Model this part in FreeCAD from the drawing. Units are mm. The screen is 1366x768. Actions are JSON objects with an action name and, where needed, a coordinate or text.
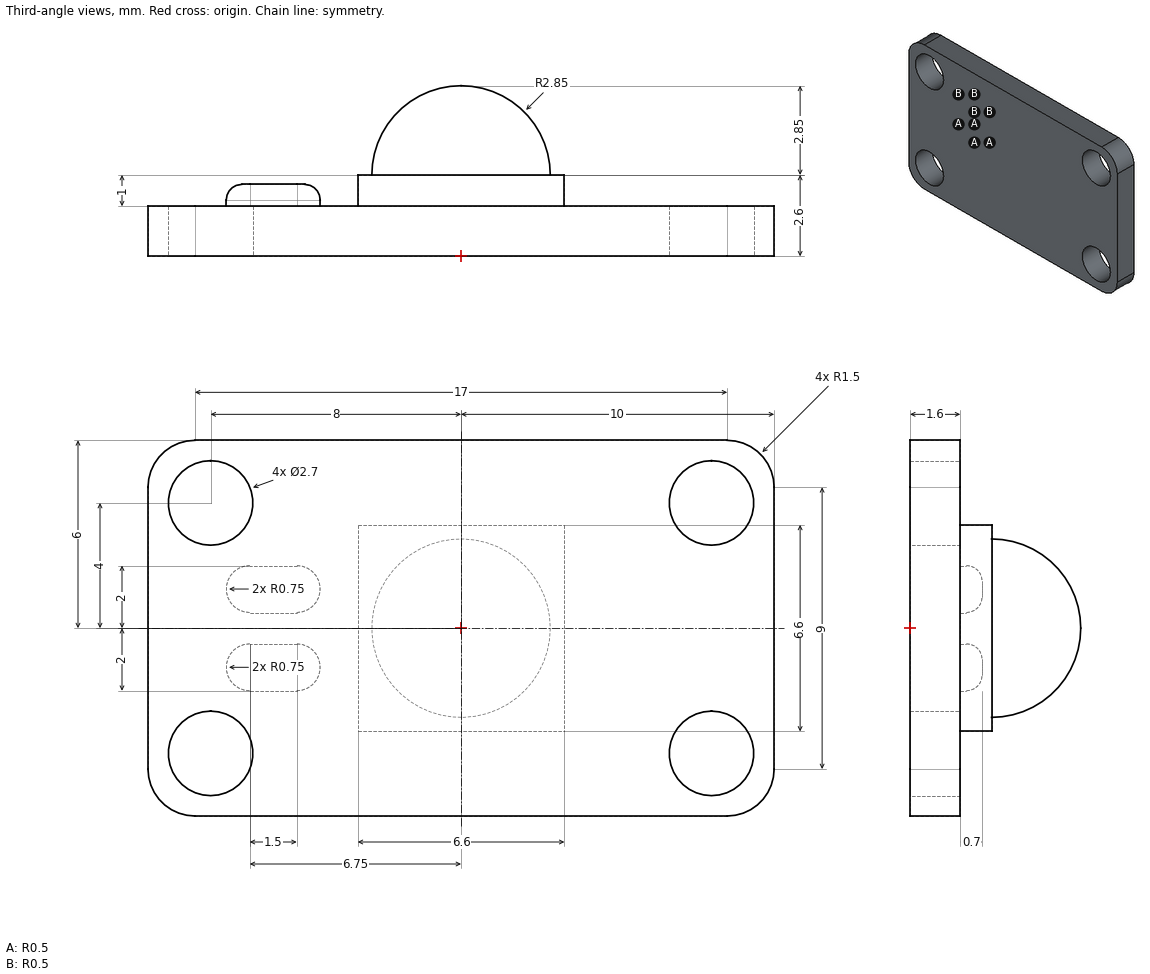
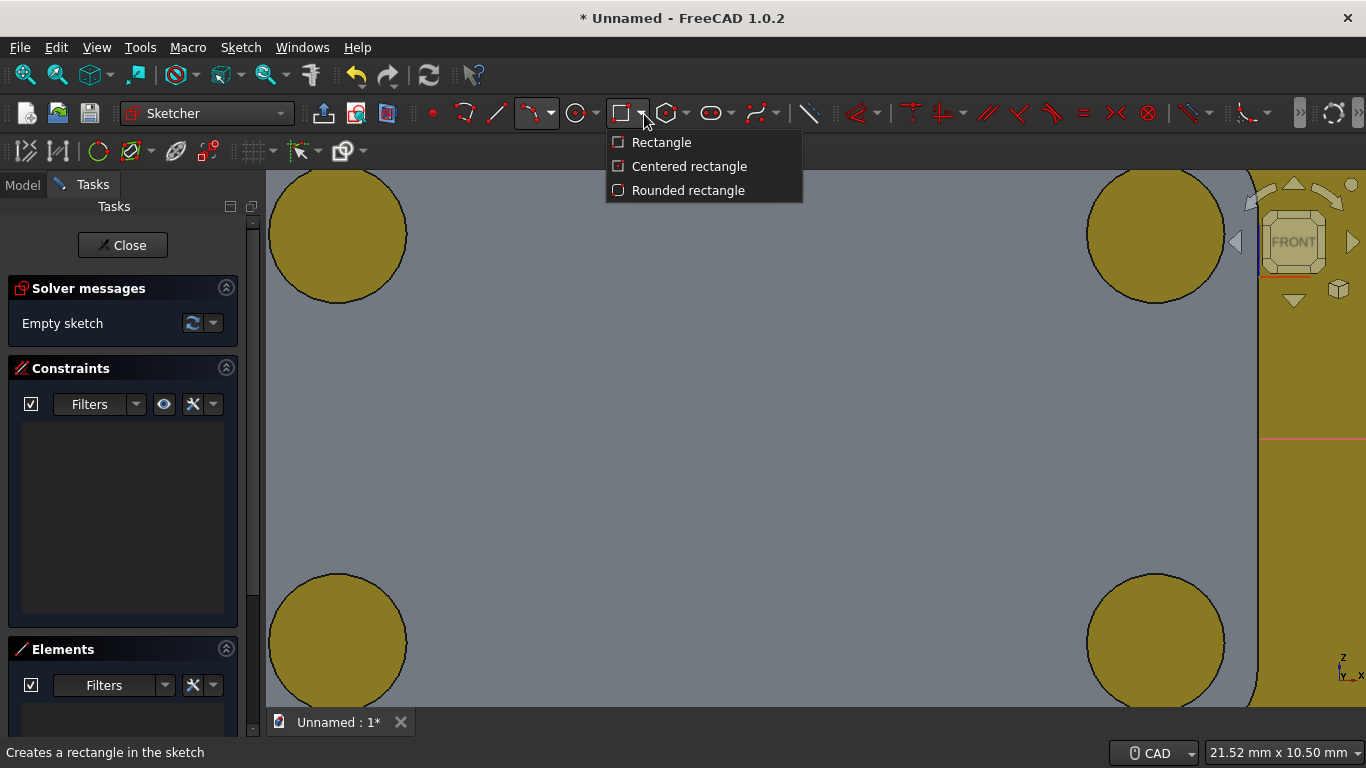
{"action": "left_click", "coordinate": [704, 166]}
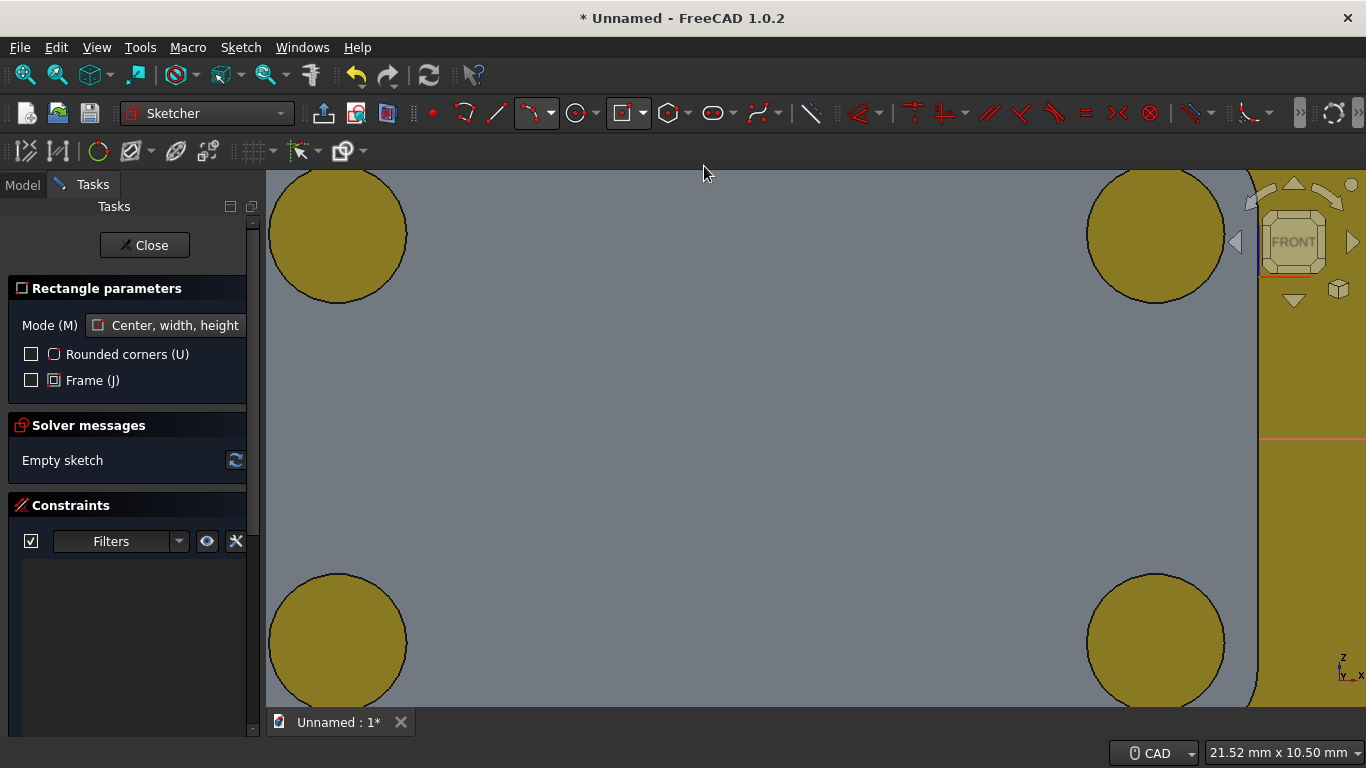
{"action": "left_click", "coordinate": [747, 438]}
{"action": "left_click", "coordinate": [915, 270]}
{"action": "key", "text": "Escape"}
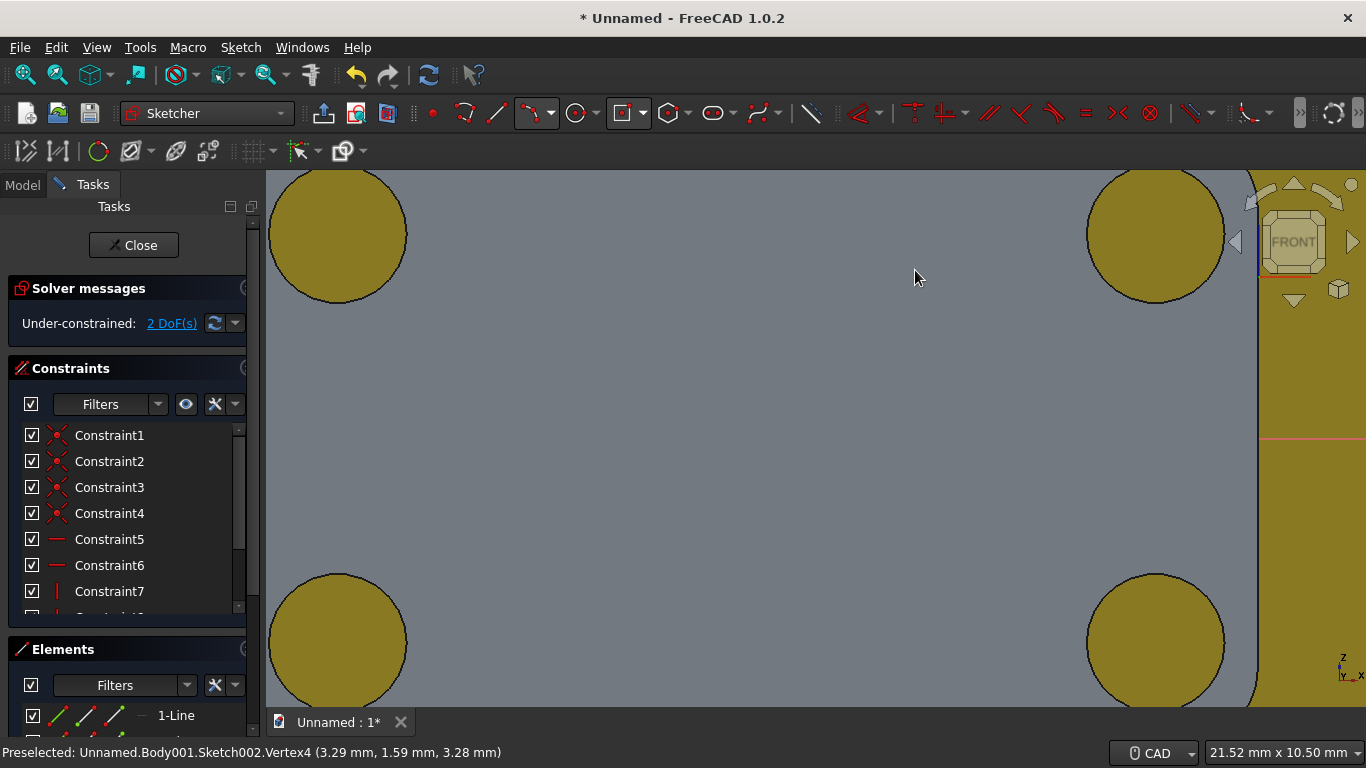
{"action": "left_click", "coordinate": [858, 114]}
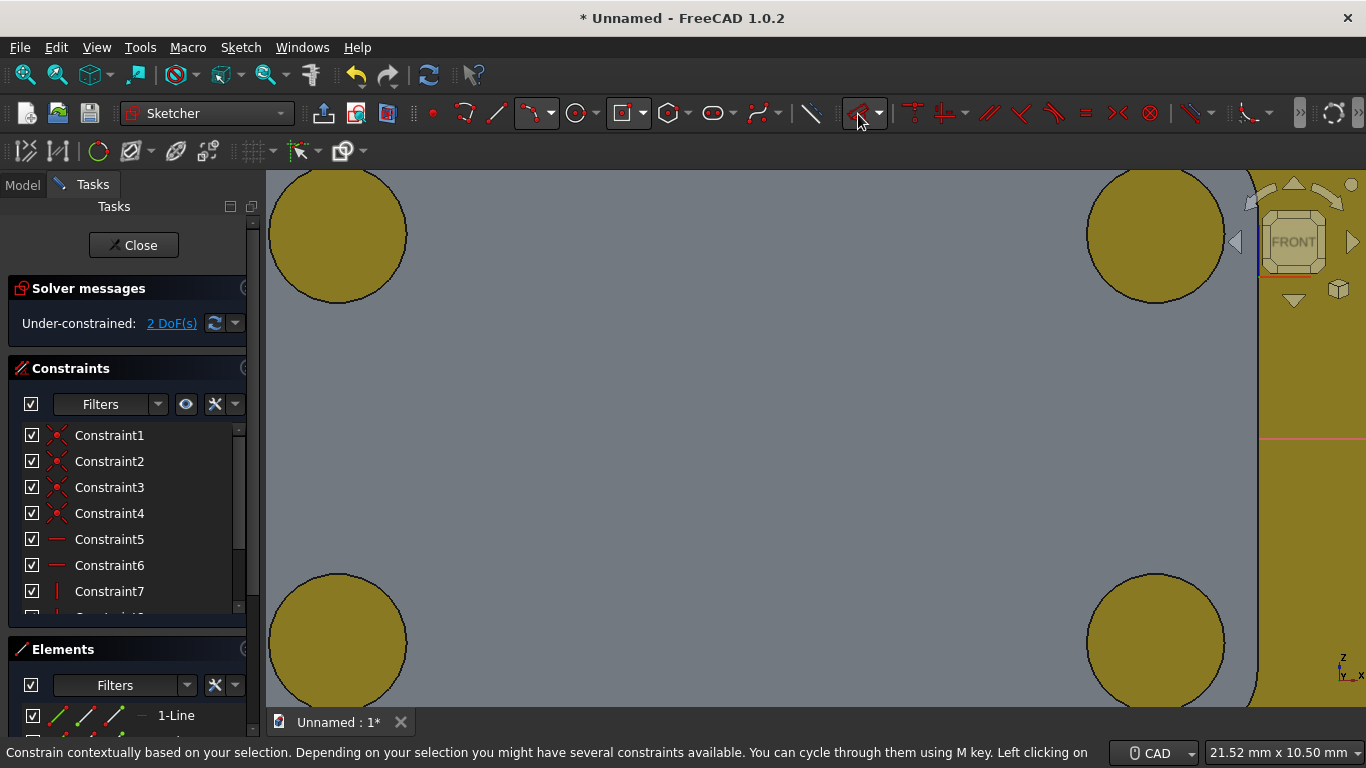
{"action": "left_click", "coordinate": [679, 606]}
{"action": "left_click", "coordinate": [669, 640]}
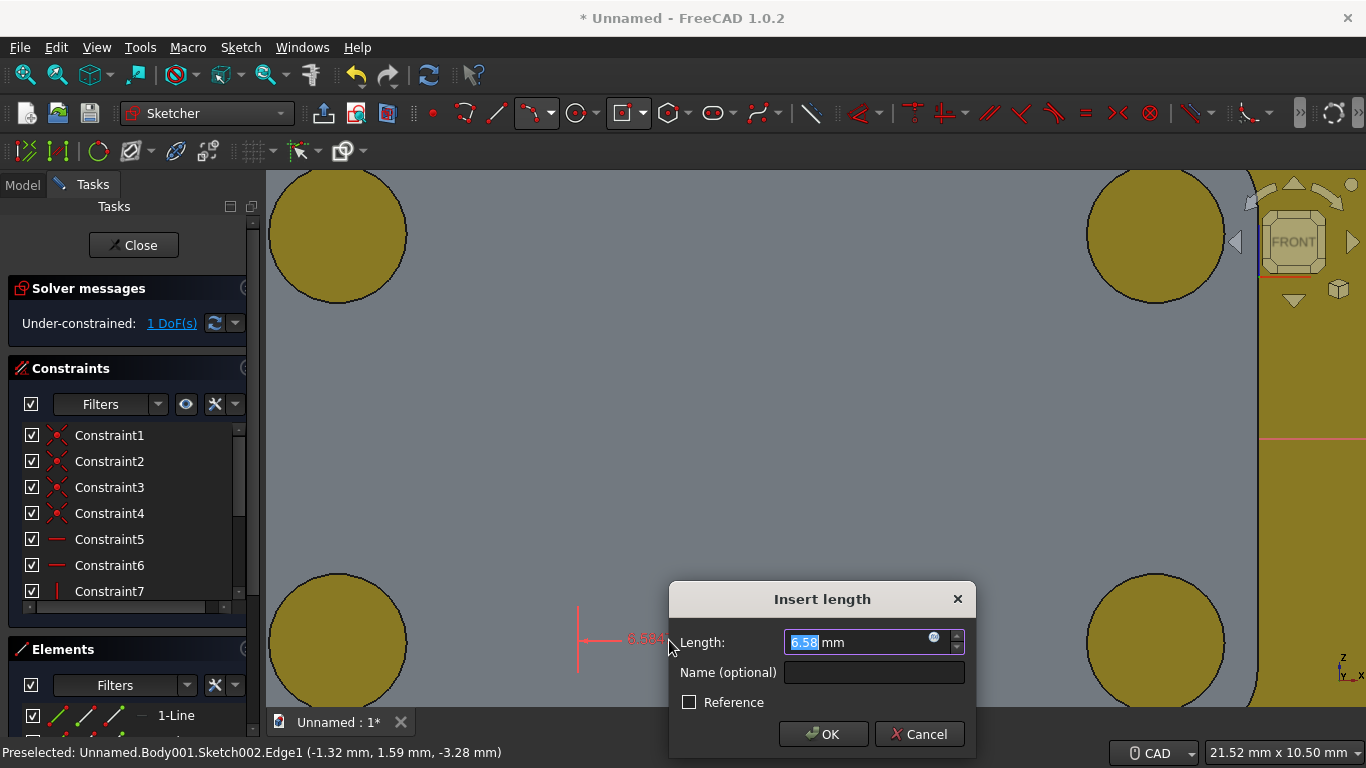
{"action": "type", "text": "6.6"}
{"action": "key", "text": "Return"}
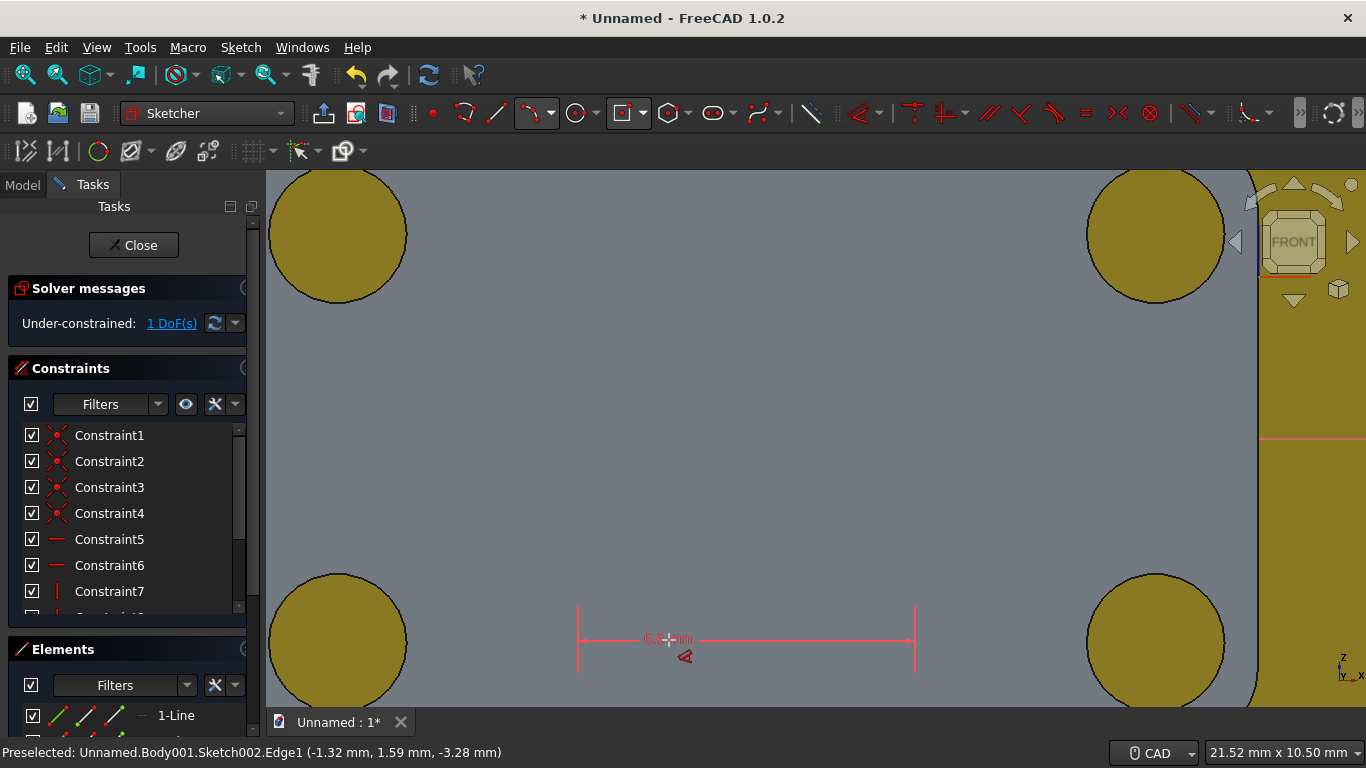
{"action": "left_click", "coordinate": [915, 506]}
{"action": "left_click", "coordinate": [949, 361]}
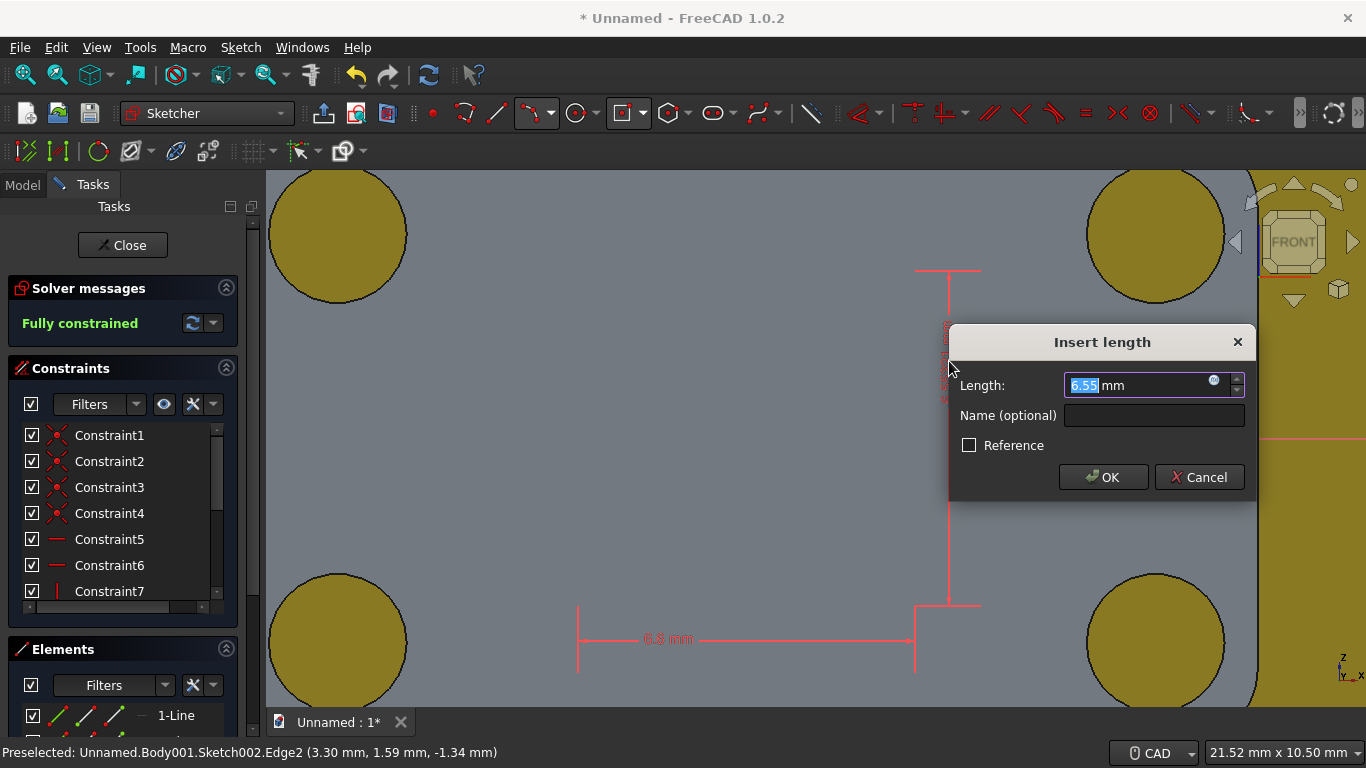
{"action": "type", "text": "6.6"}
{"action": "key", "text": "Return"}
{"action": "key", "text": "Escape"}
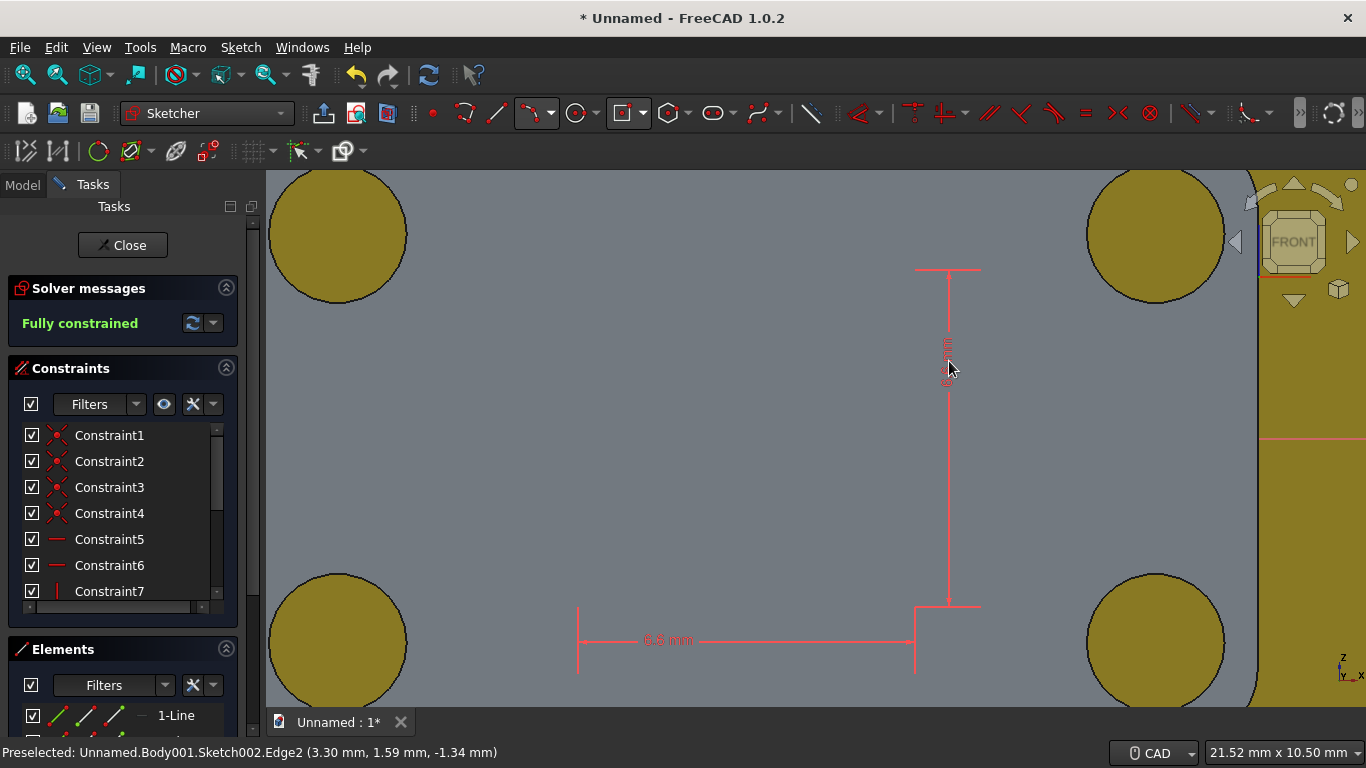
{"action": "left_click", "coordinate": [123, 245]}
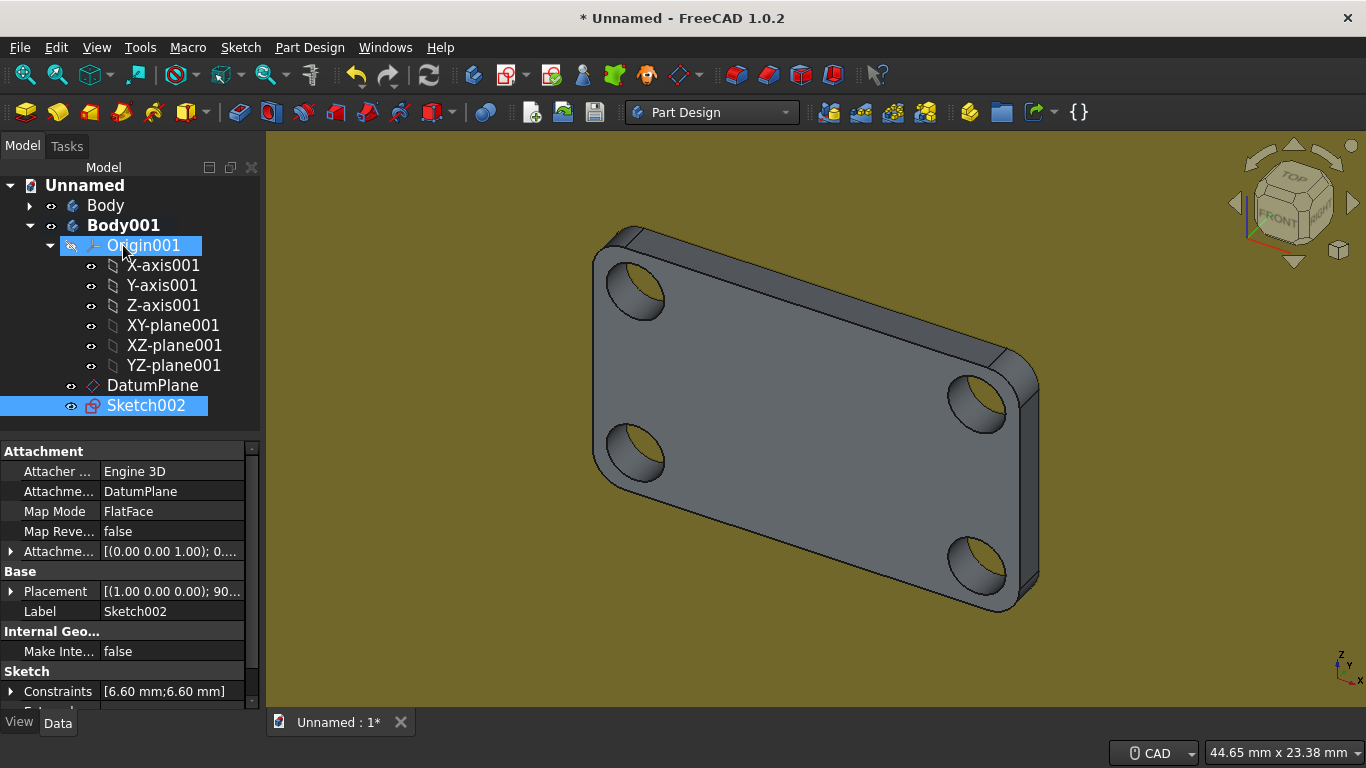
{"action": "left_click", "coordinate": [26, 112]}